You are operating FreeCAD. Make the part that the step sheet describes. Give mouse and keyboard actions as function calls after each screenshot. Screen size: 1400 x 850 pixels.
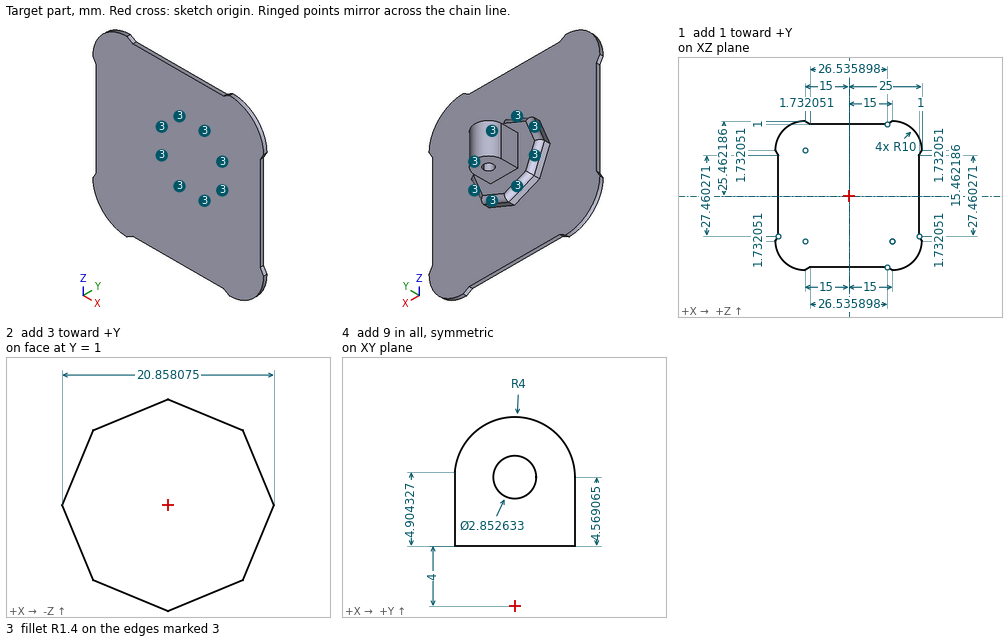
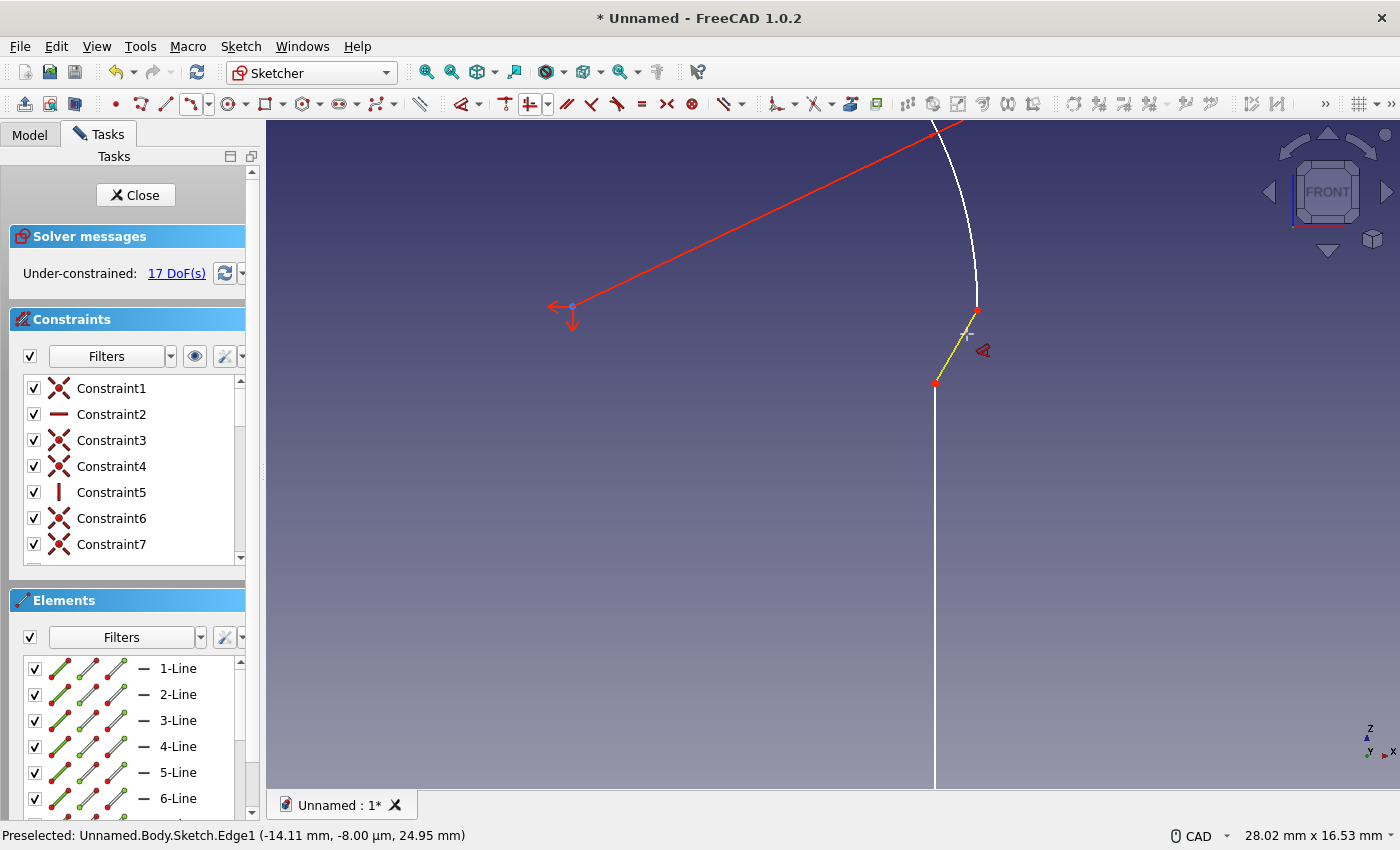
click(965, 332)
click(956, 276)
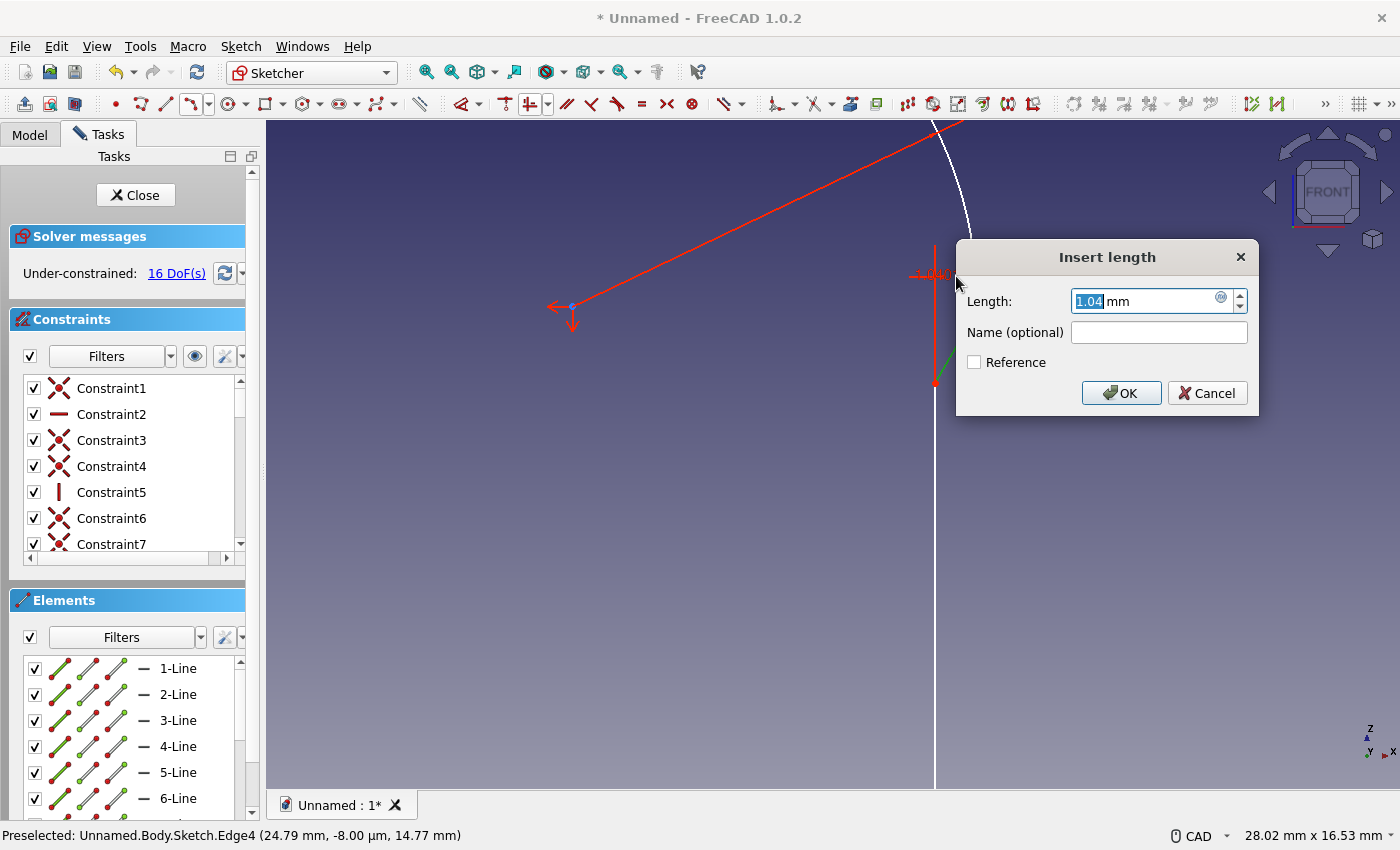
text(1)
key(Return)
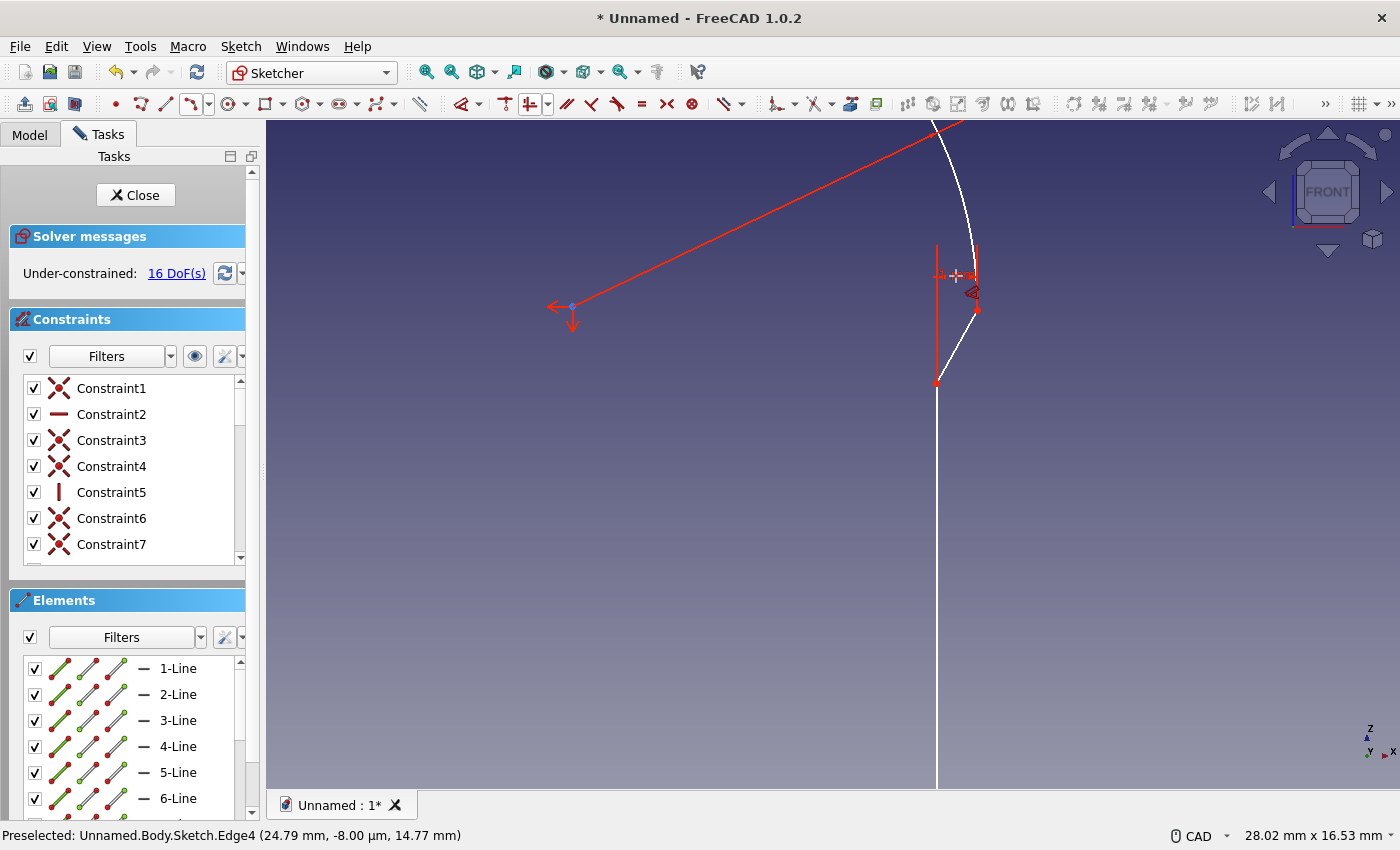
scroll(968, 334, down, 8)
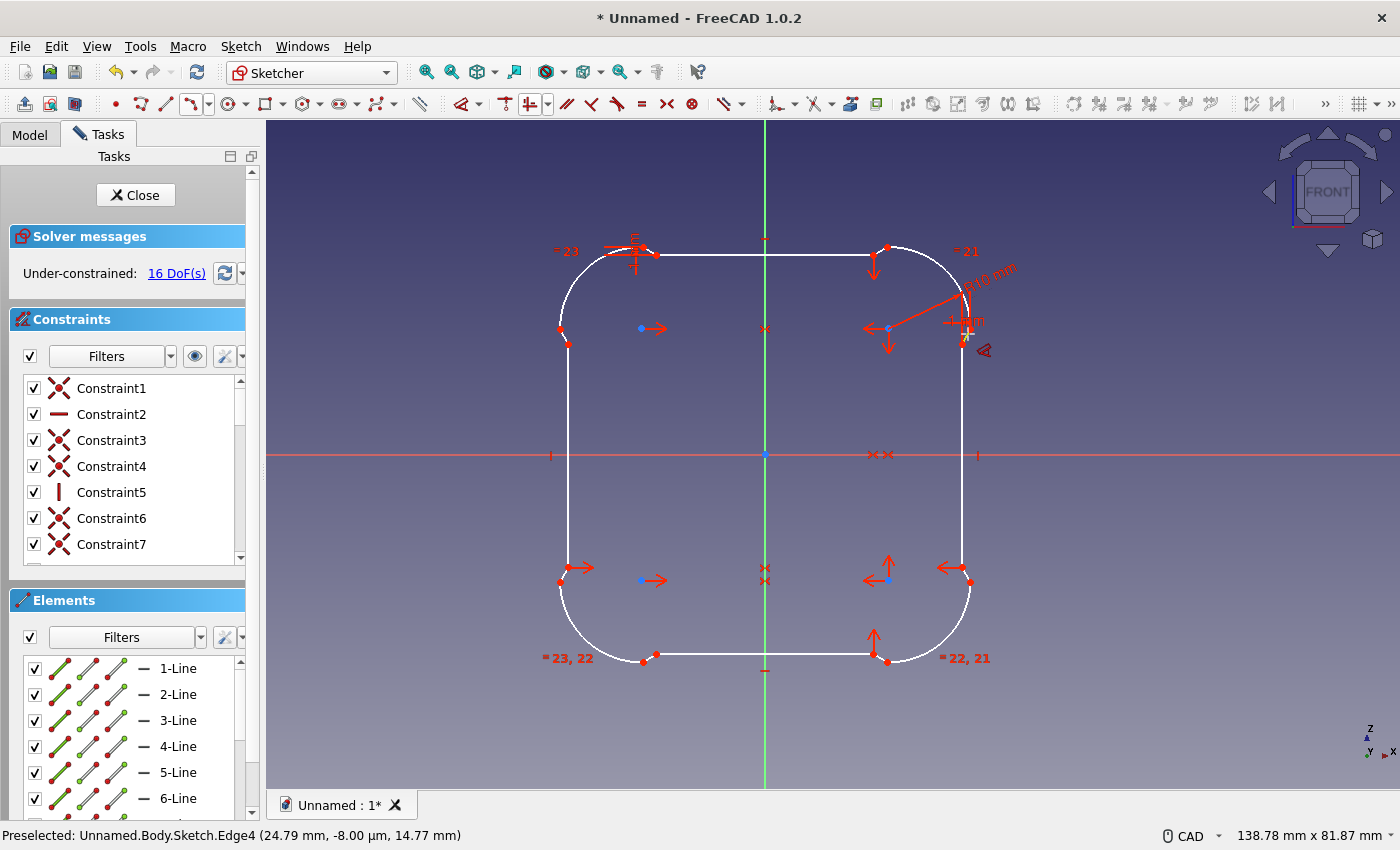
click(643, 247)
click(704, 213)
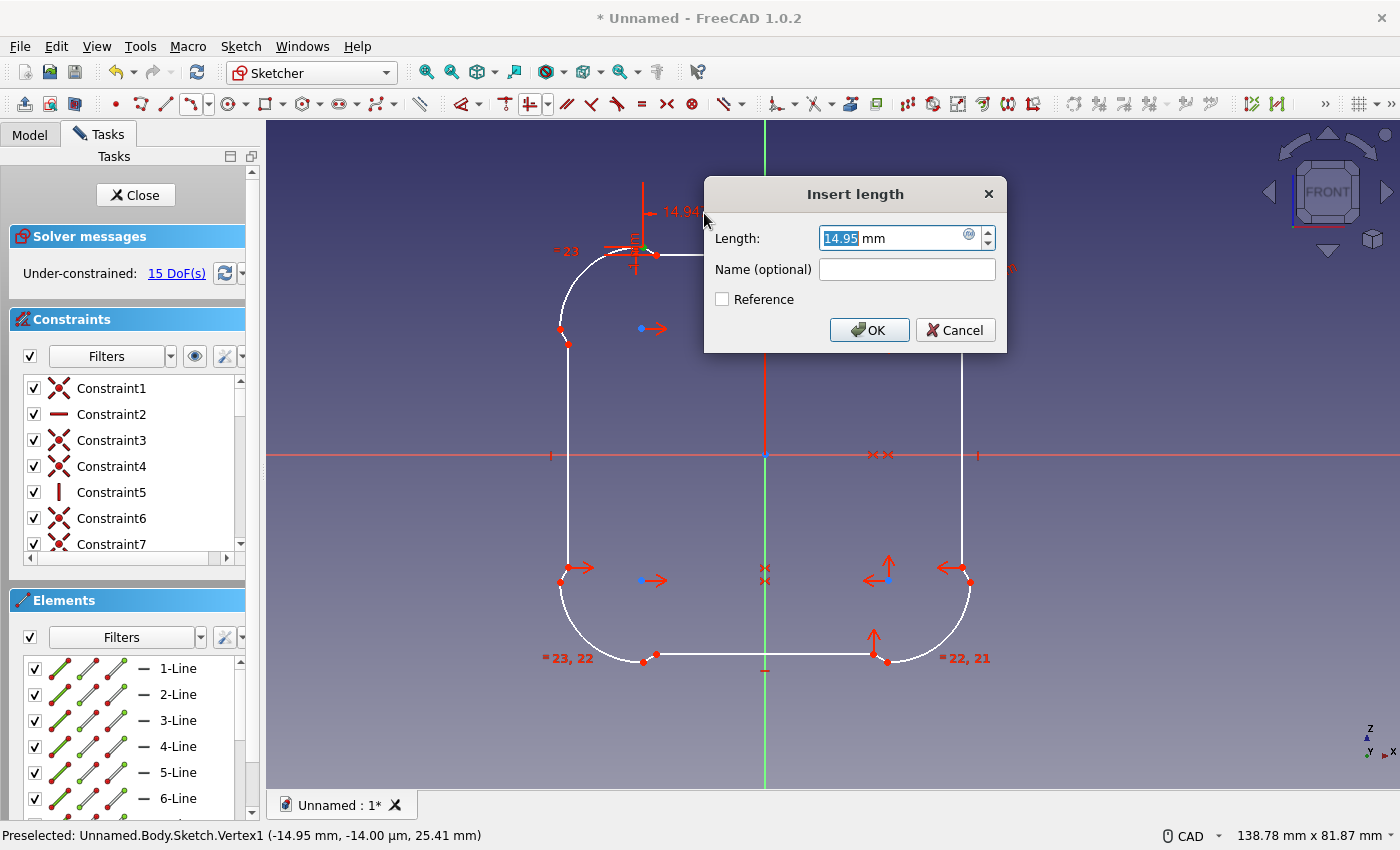
text(15)
key(Return)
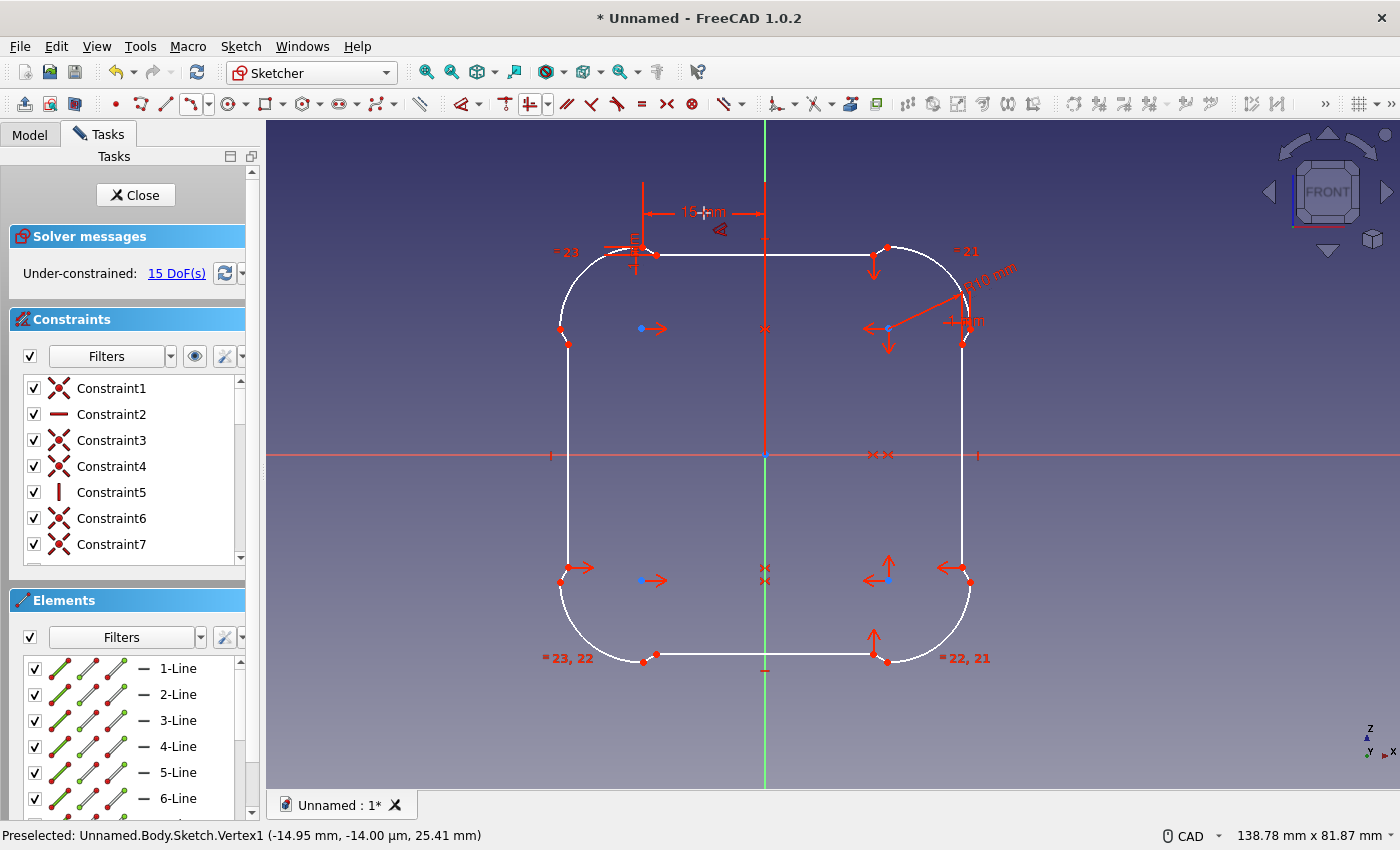
click(887, 247)
click(826, 213)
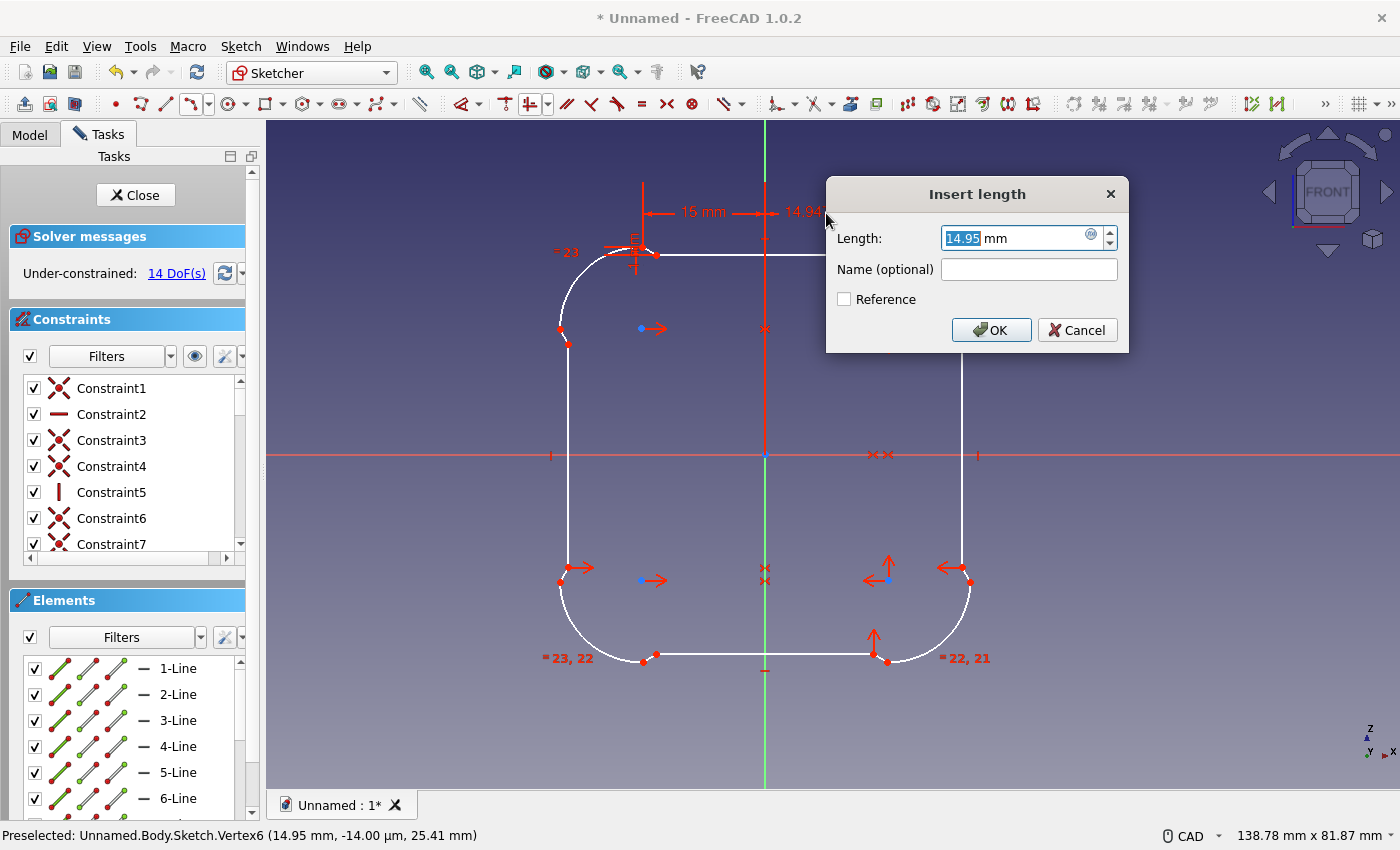
text(15)
key(Return)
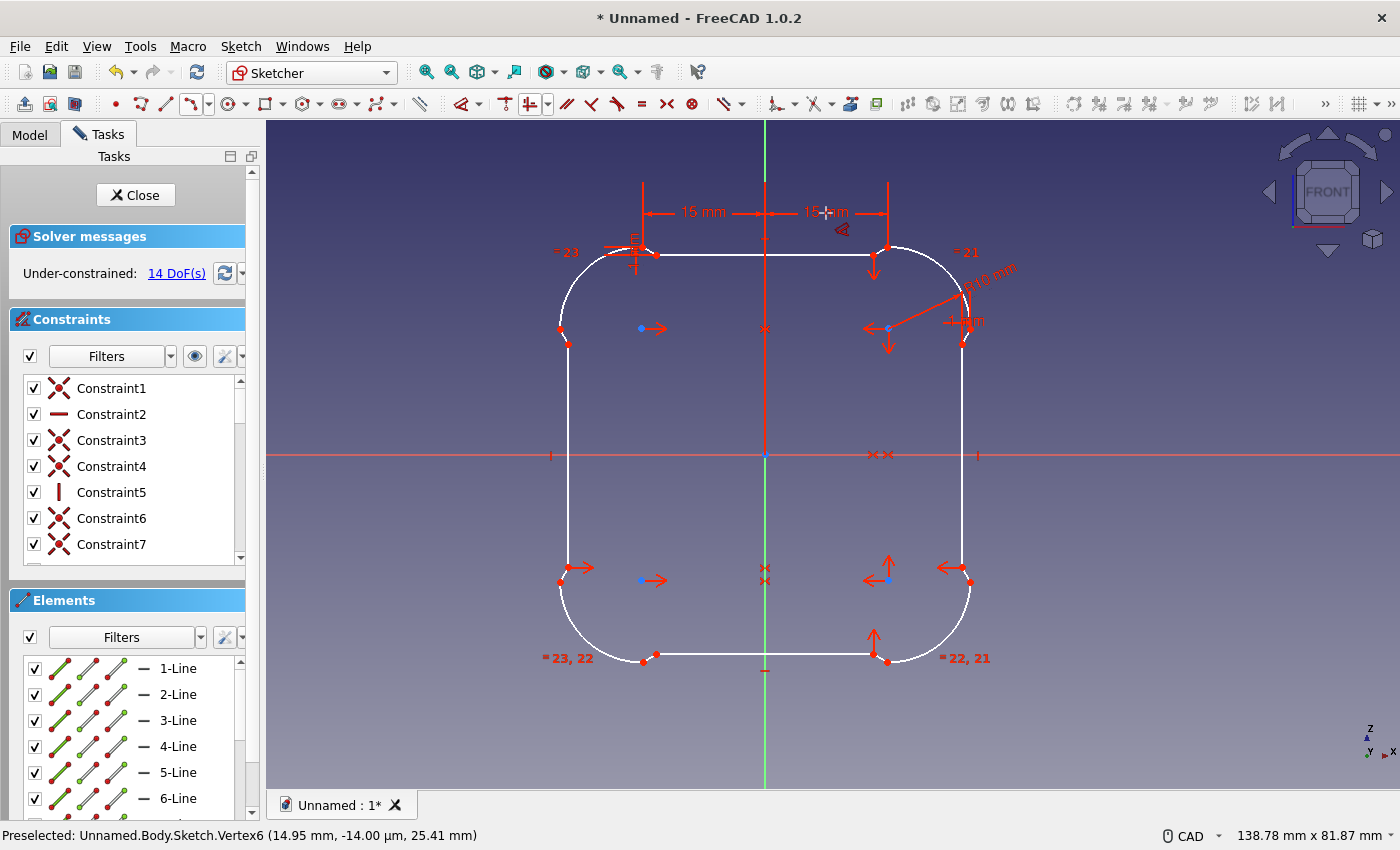
click(970, 330)
click(868, 296)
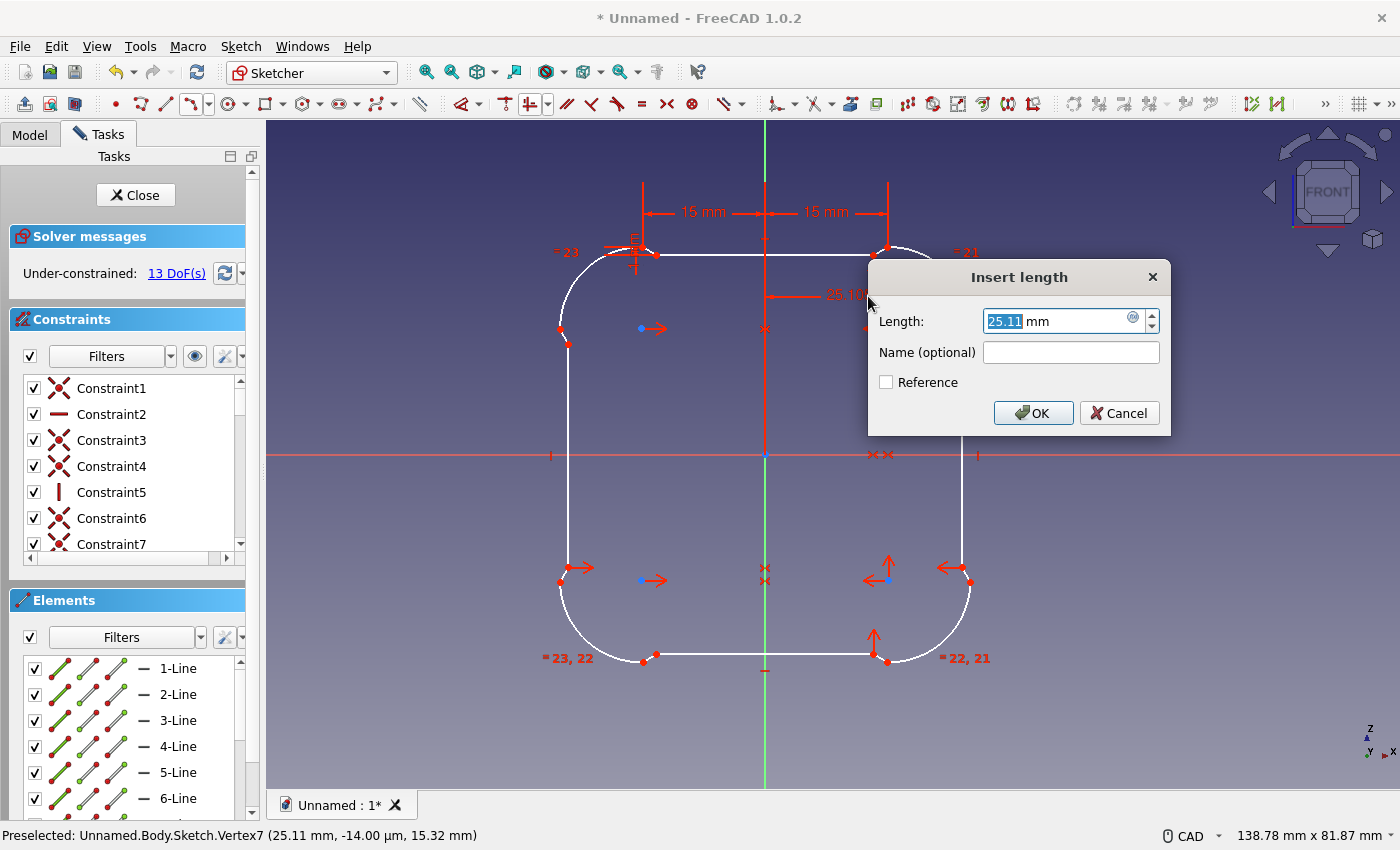
text(25)
key(Return)